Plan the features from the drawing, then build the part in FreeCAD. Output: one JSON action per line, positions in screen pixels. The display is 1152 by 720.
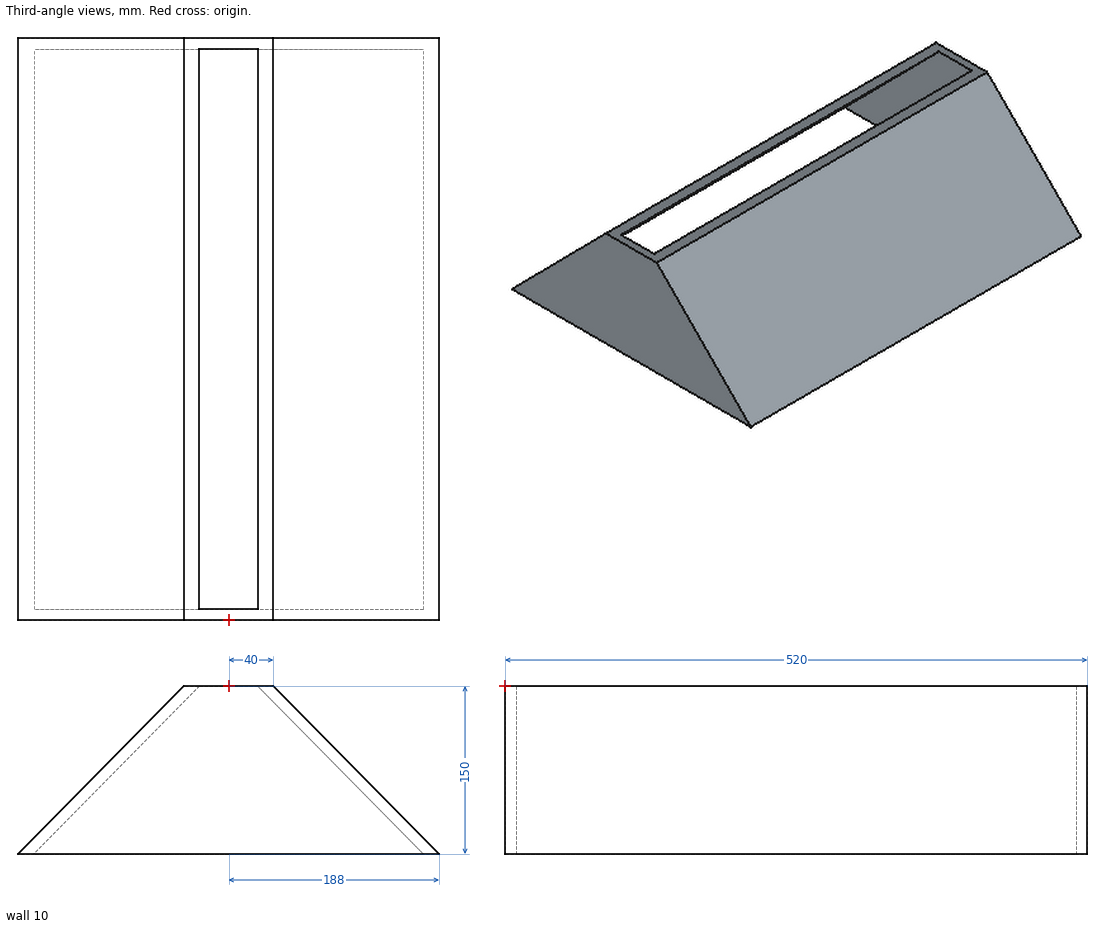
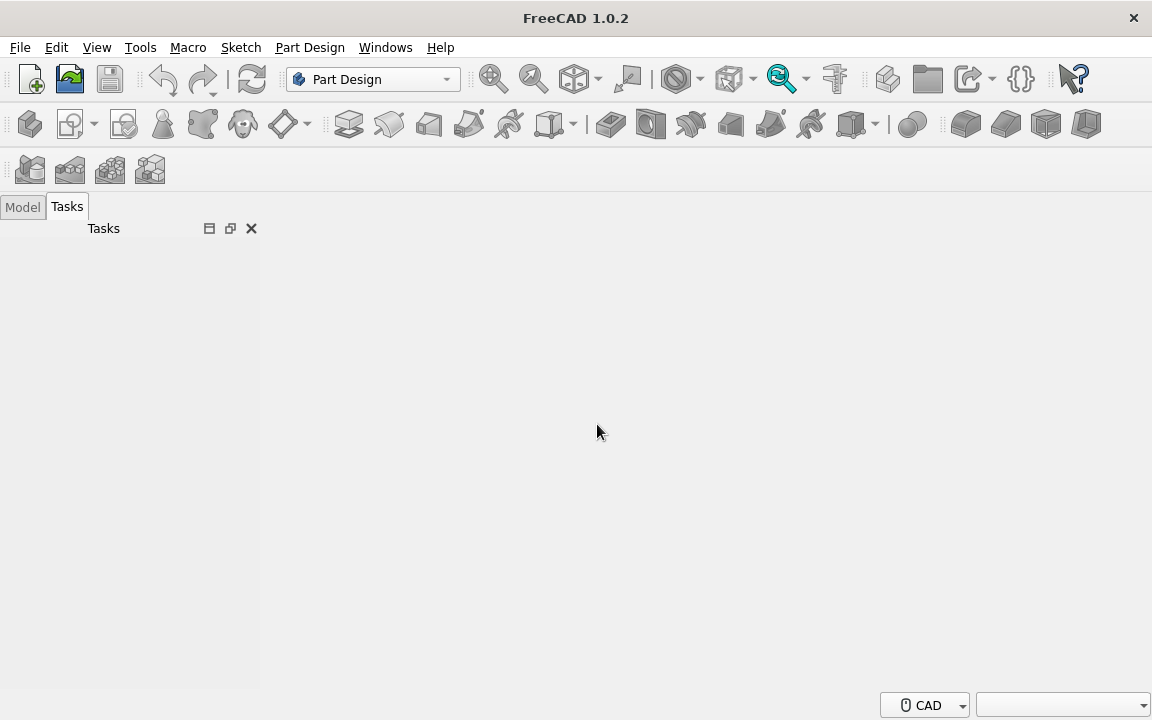
{"action": "key", "text": "ctrl+n"}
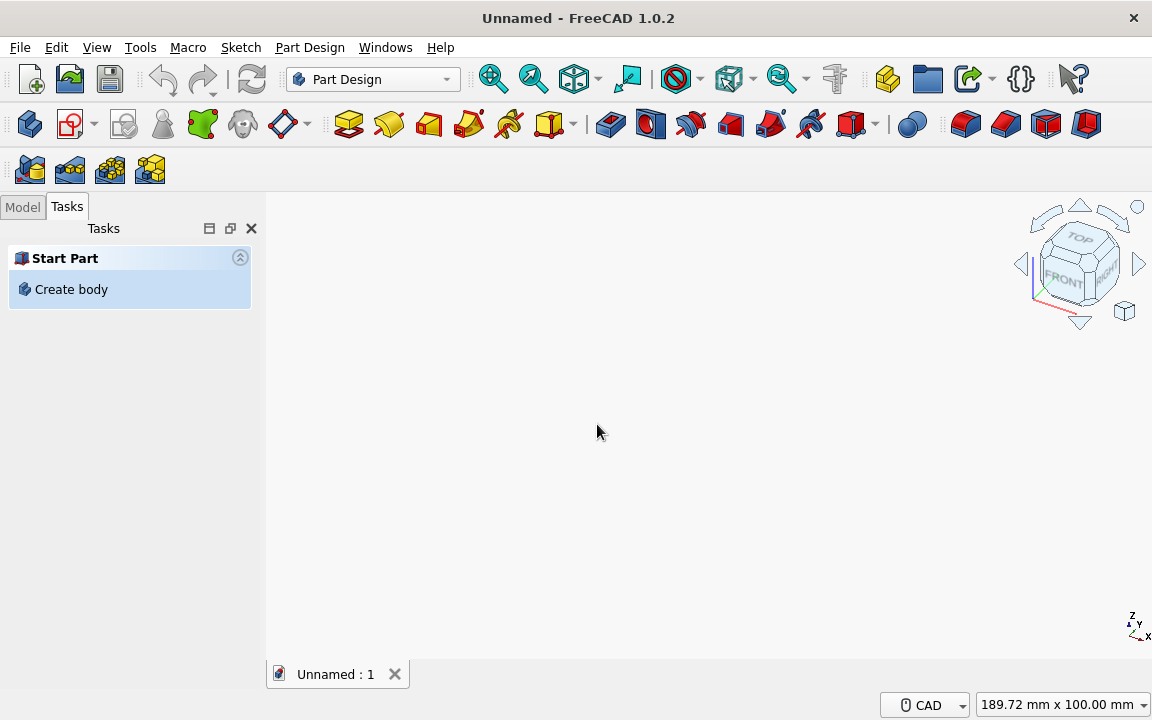
{"action": "left_click", "coordinate": [70, 124]}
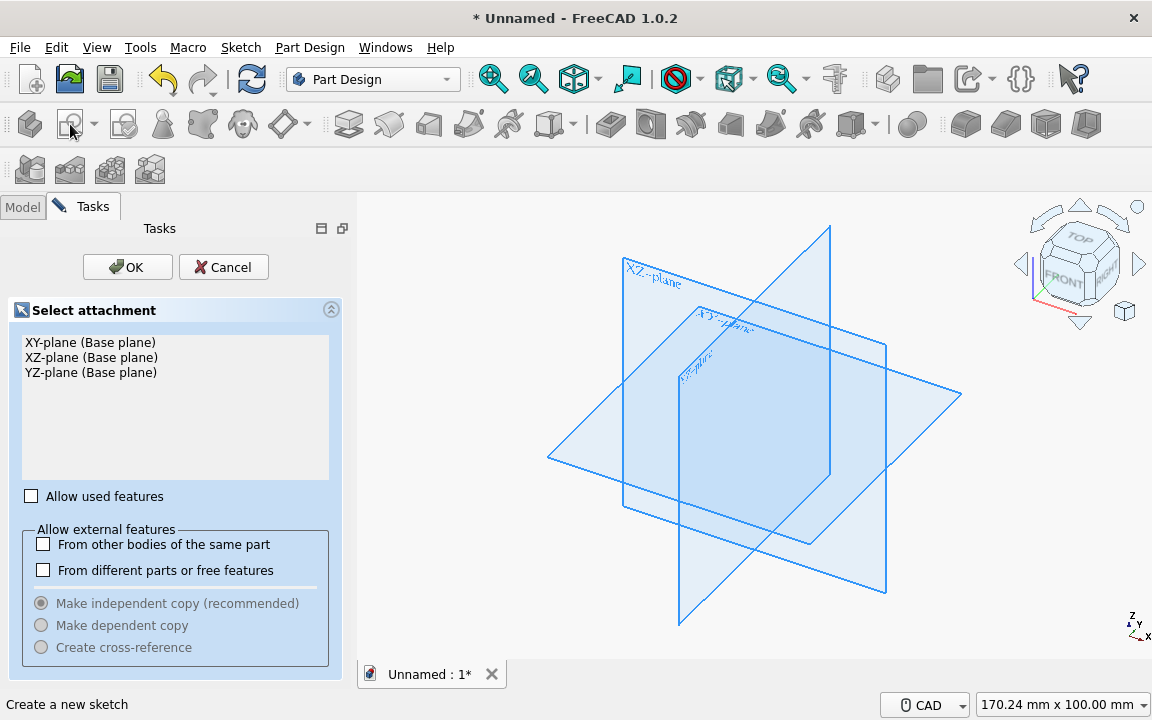
{"action": "left_click", "coordinate": [82, 358]}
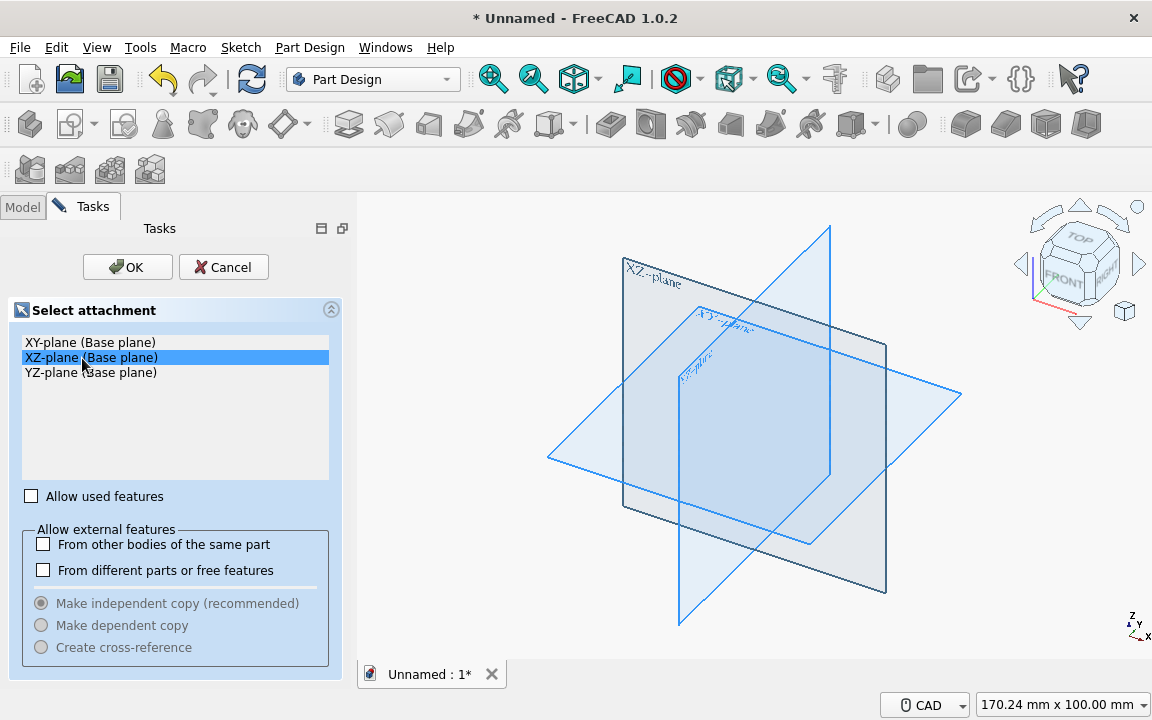
{"action": "left_click", "coordinate": [128, 267]}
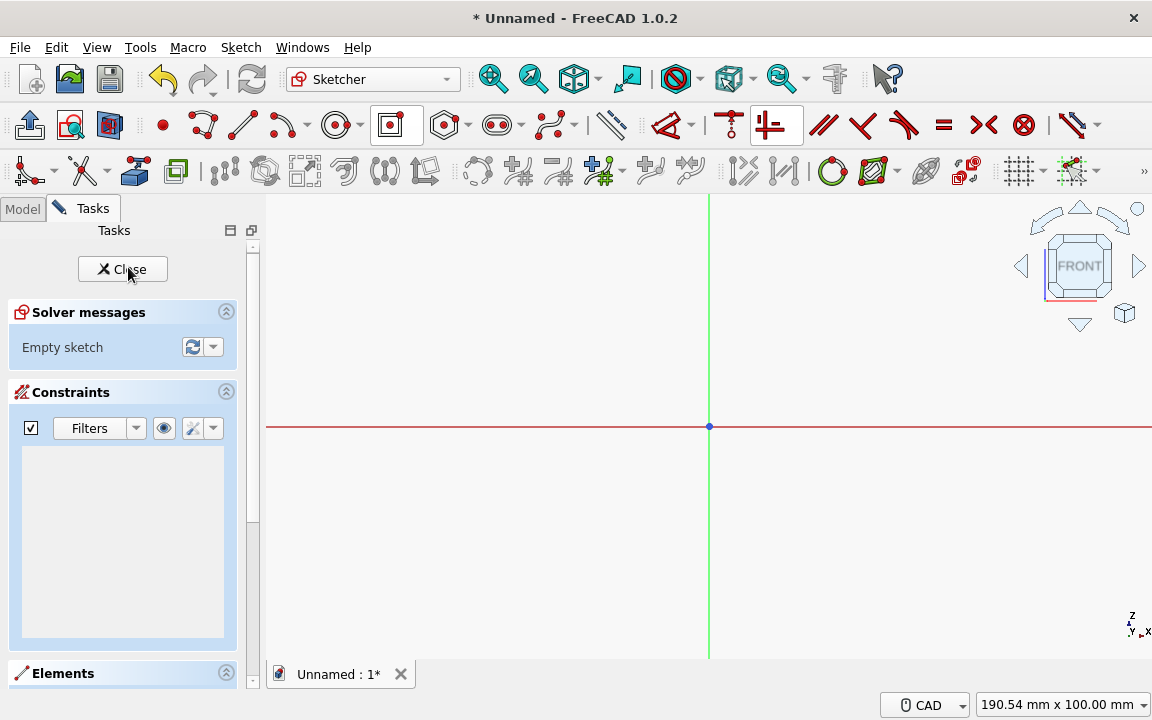
{"action": "scroll", "coordinate": [346, 224], "scroll_direction": "down", "scroll_amount": 5}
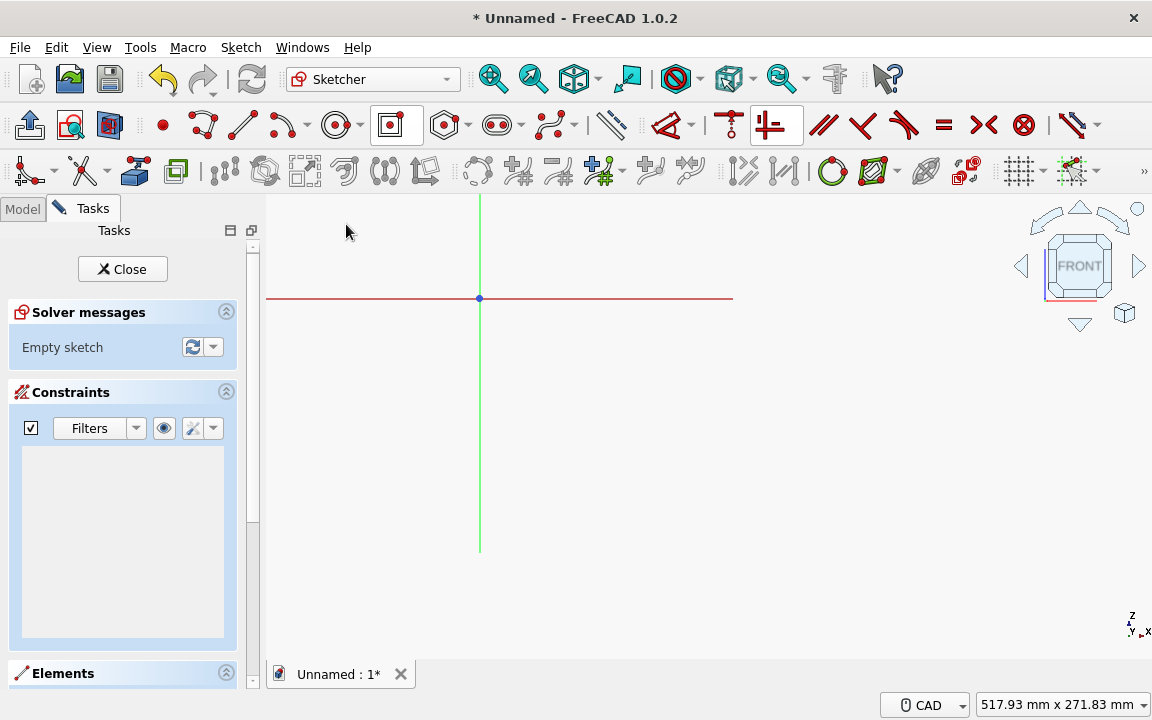
{"action": "key", "text": "g m"}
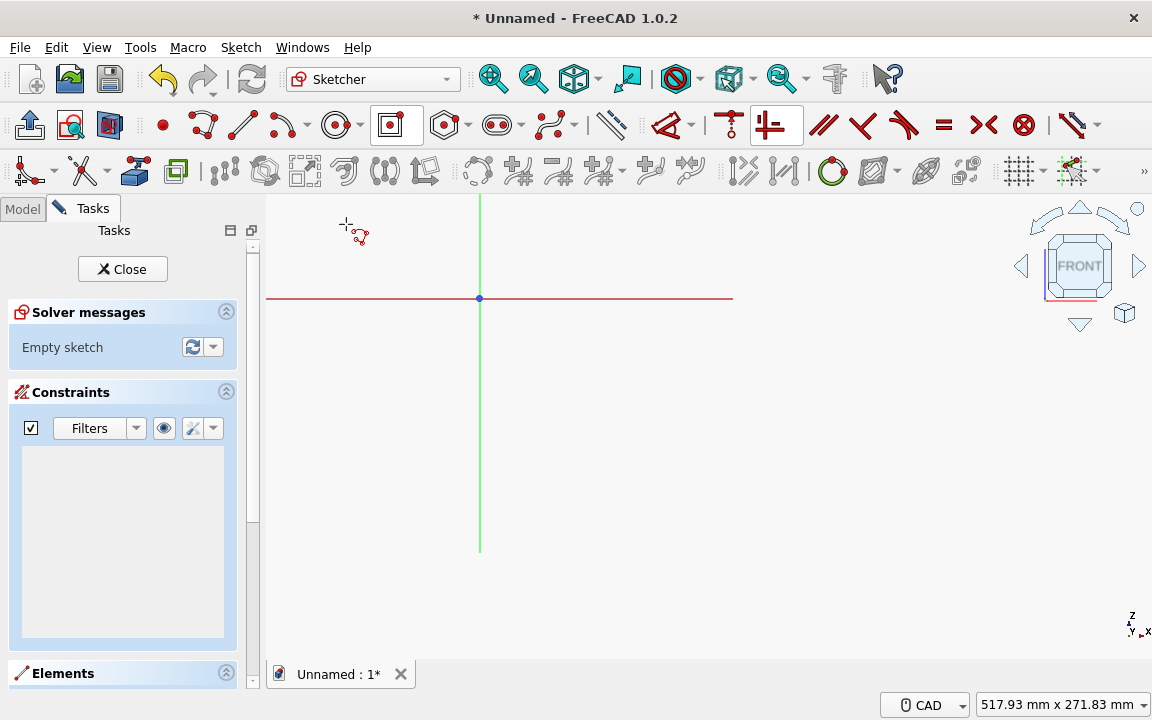
{"action": "left_click", "coordinate": [480, 299]}
{"action": "left_click", "coordinate": [548, 308]}
{"action": "left_click", "coordinate": [801, 555]}
{"action": "left_click", "coordinate": [489, 555]}
{"action": "left_click", "coordinate": [480, 299]}
{"action": "key", "text": "Escape"}
{"action": "key", "text": "Escape"}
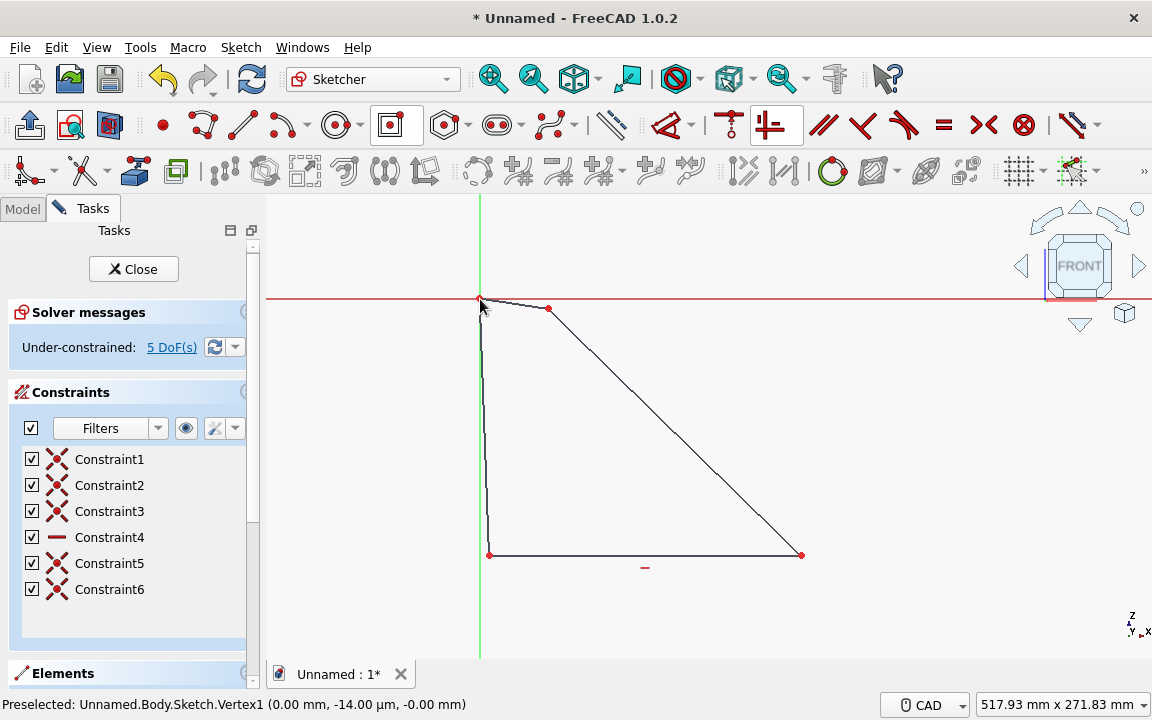
{"action": "left_click", "coordinate": [500, 302]}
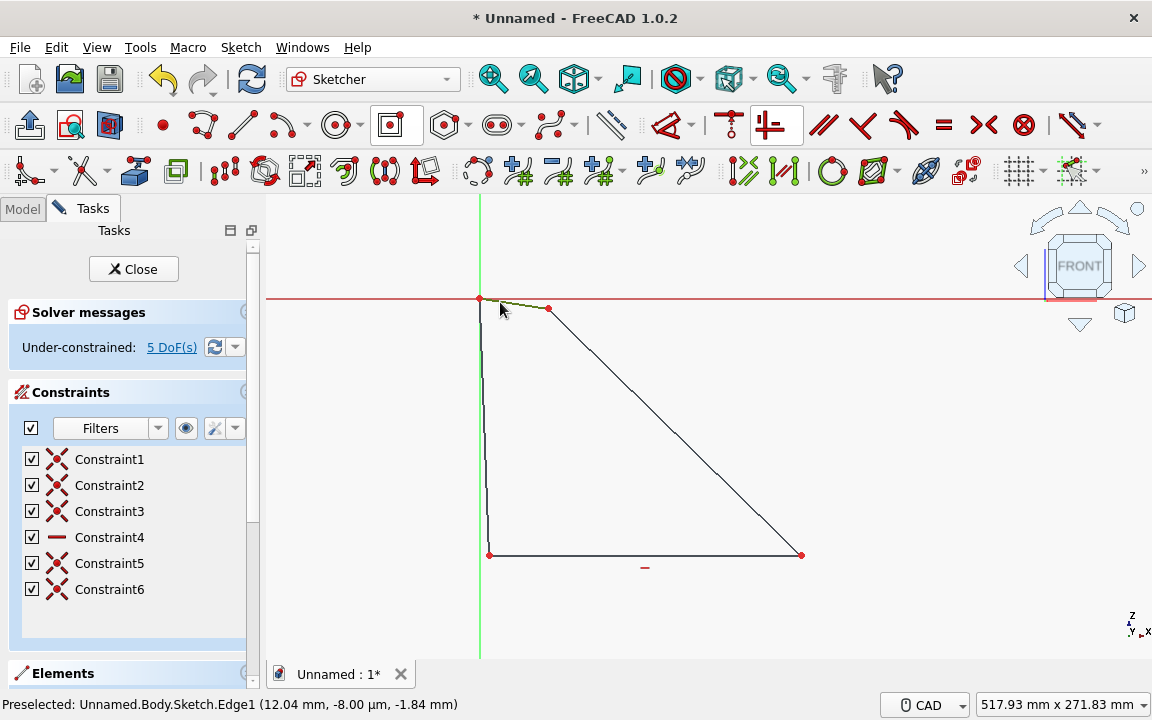
{"action": "key", "text": "h"}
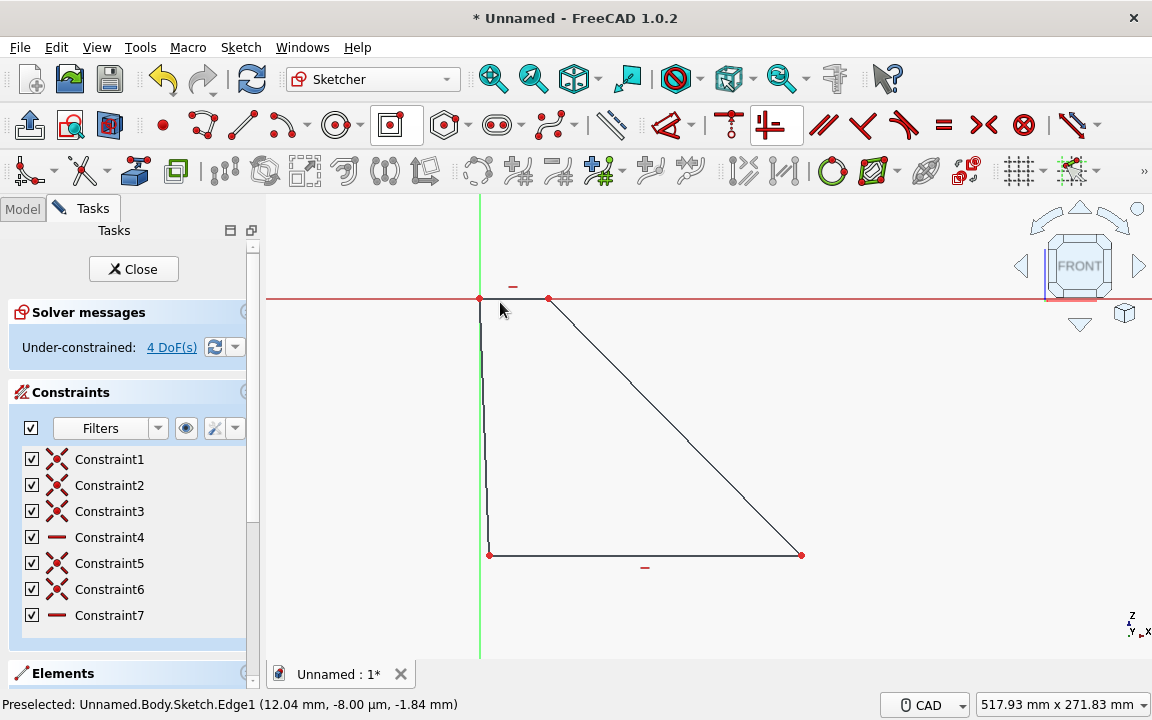
{"action": "left_click", "coordinate": [482, 376]}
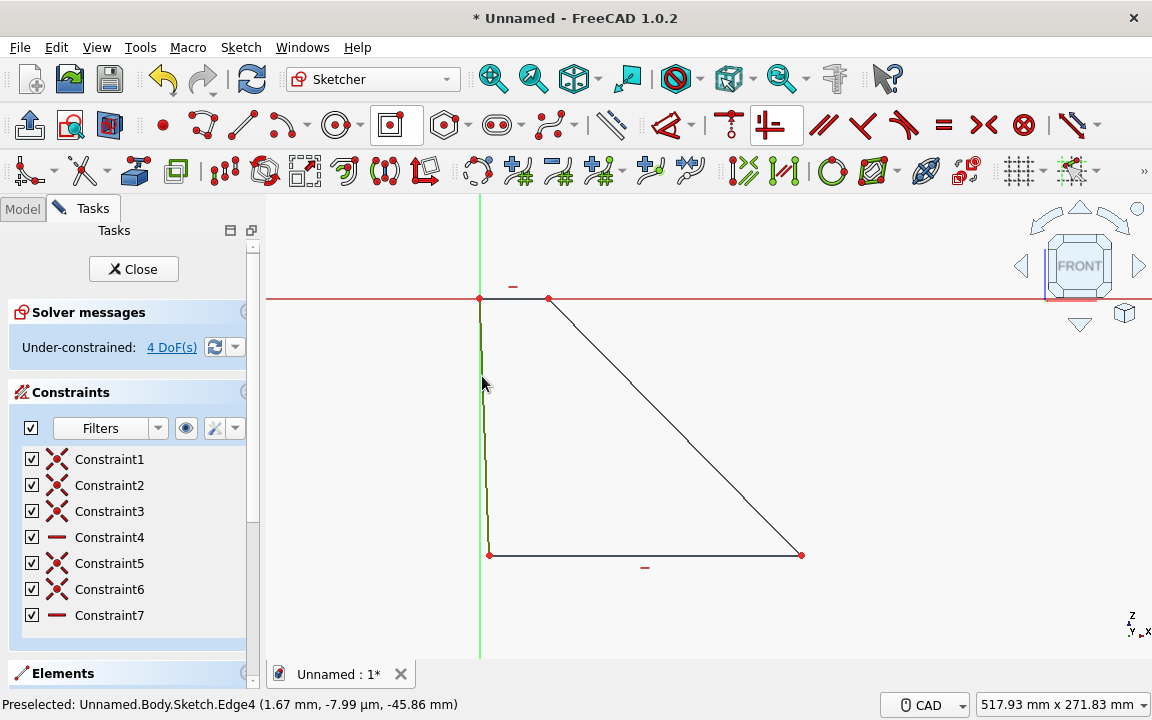
{"action": "key", "text": "v"}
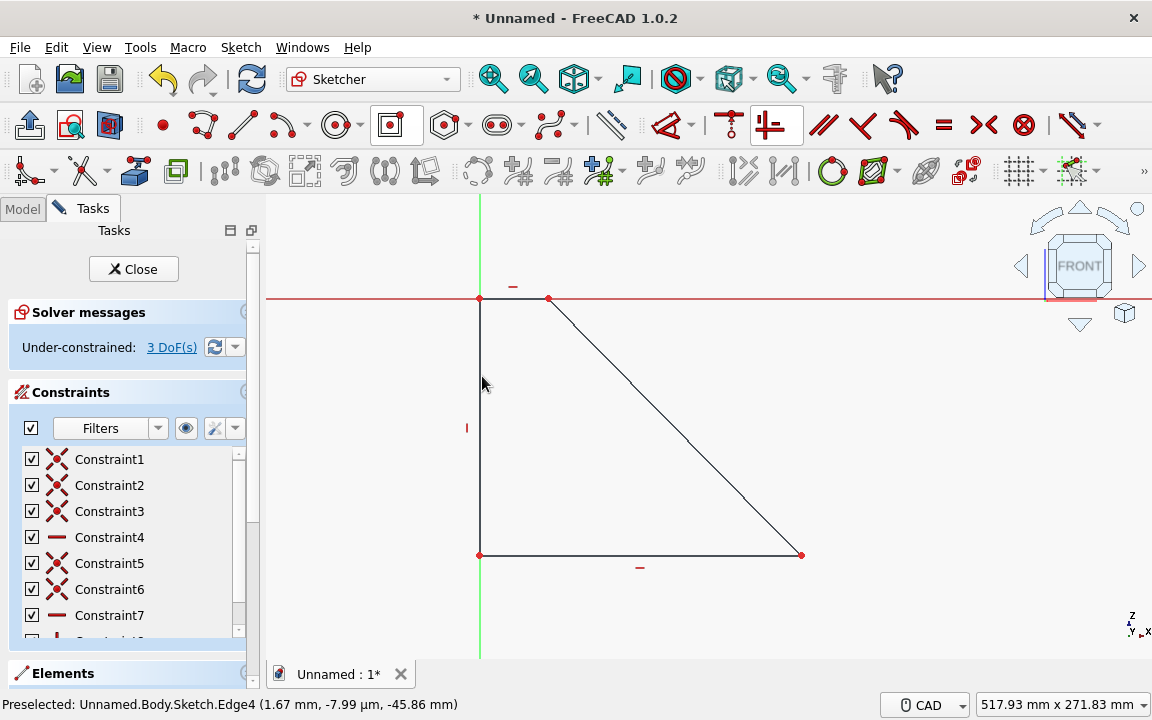
{"action": "key", "text": "d"}